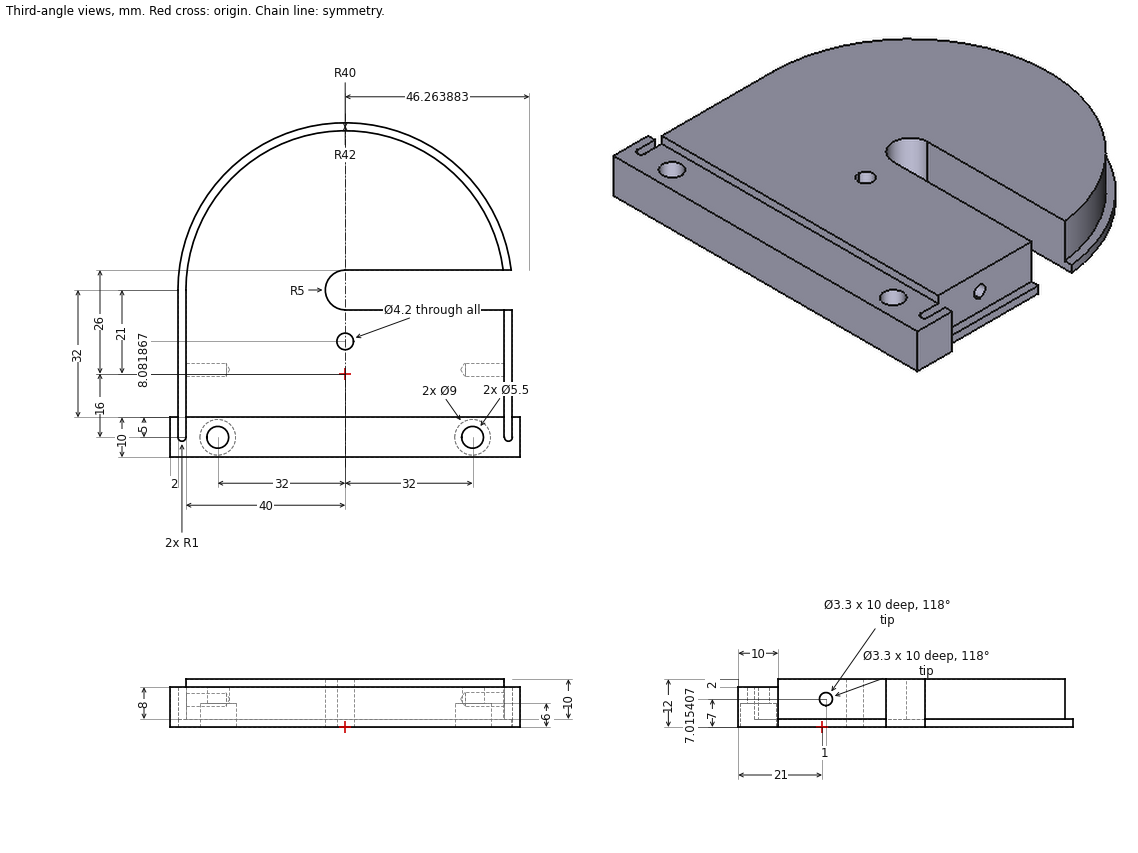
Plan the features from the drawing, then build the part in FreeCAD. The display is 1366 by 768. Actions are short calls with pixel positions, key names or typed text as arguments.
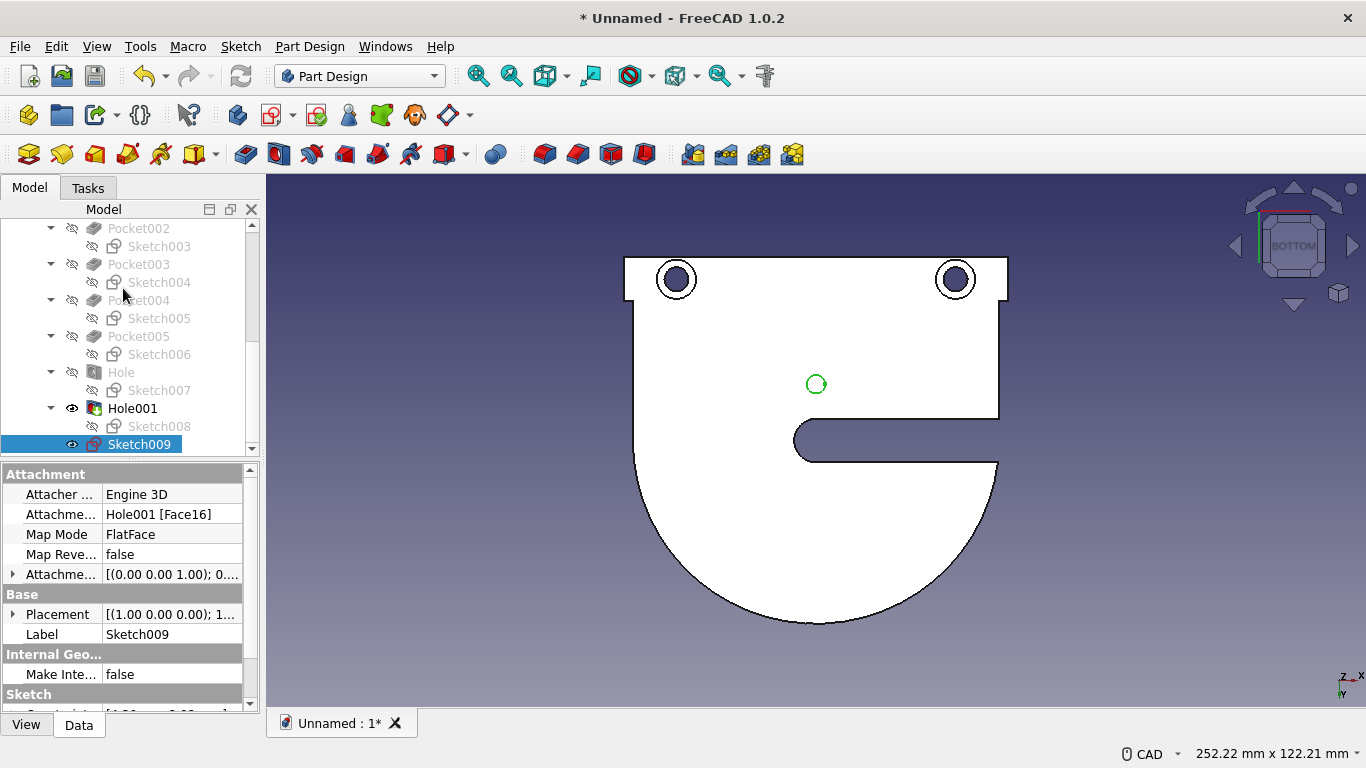
click(279, 154)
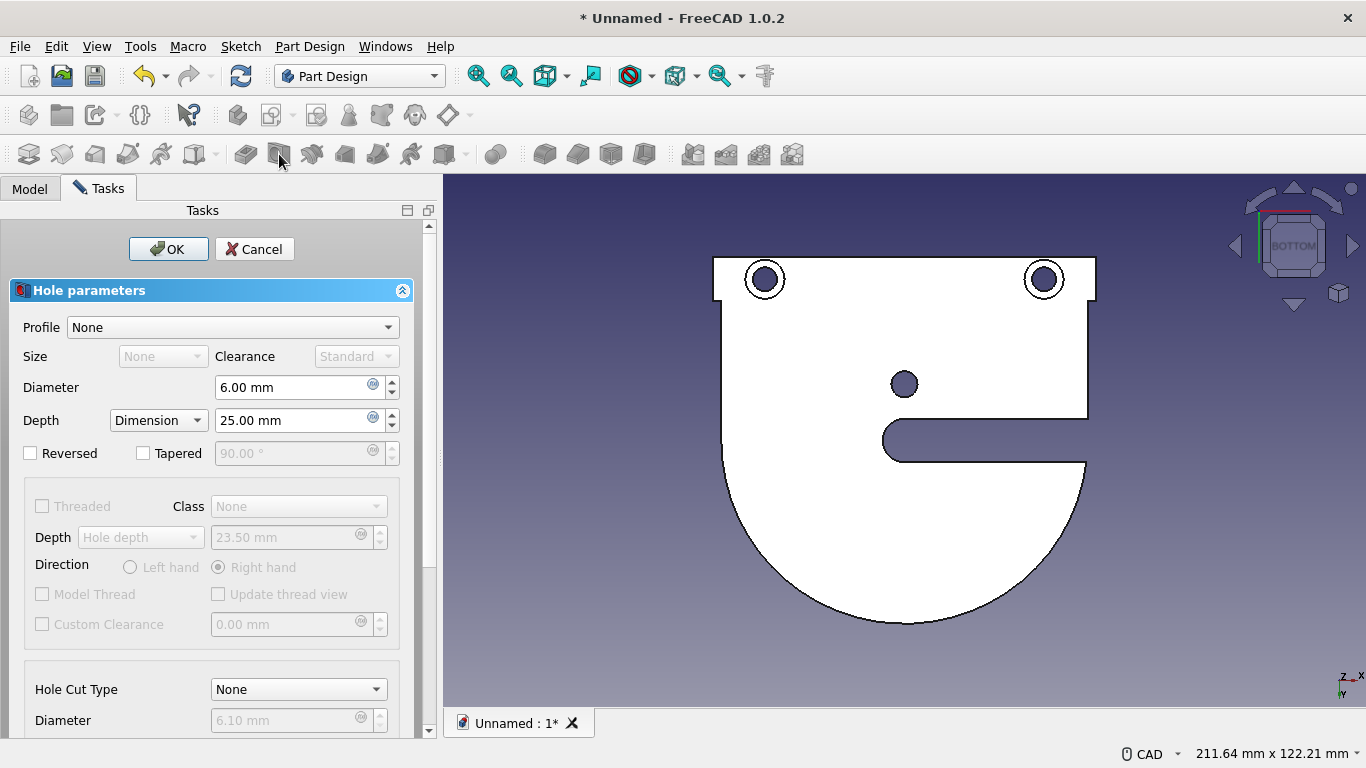
triple_click(300, 388)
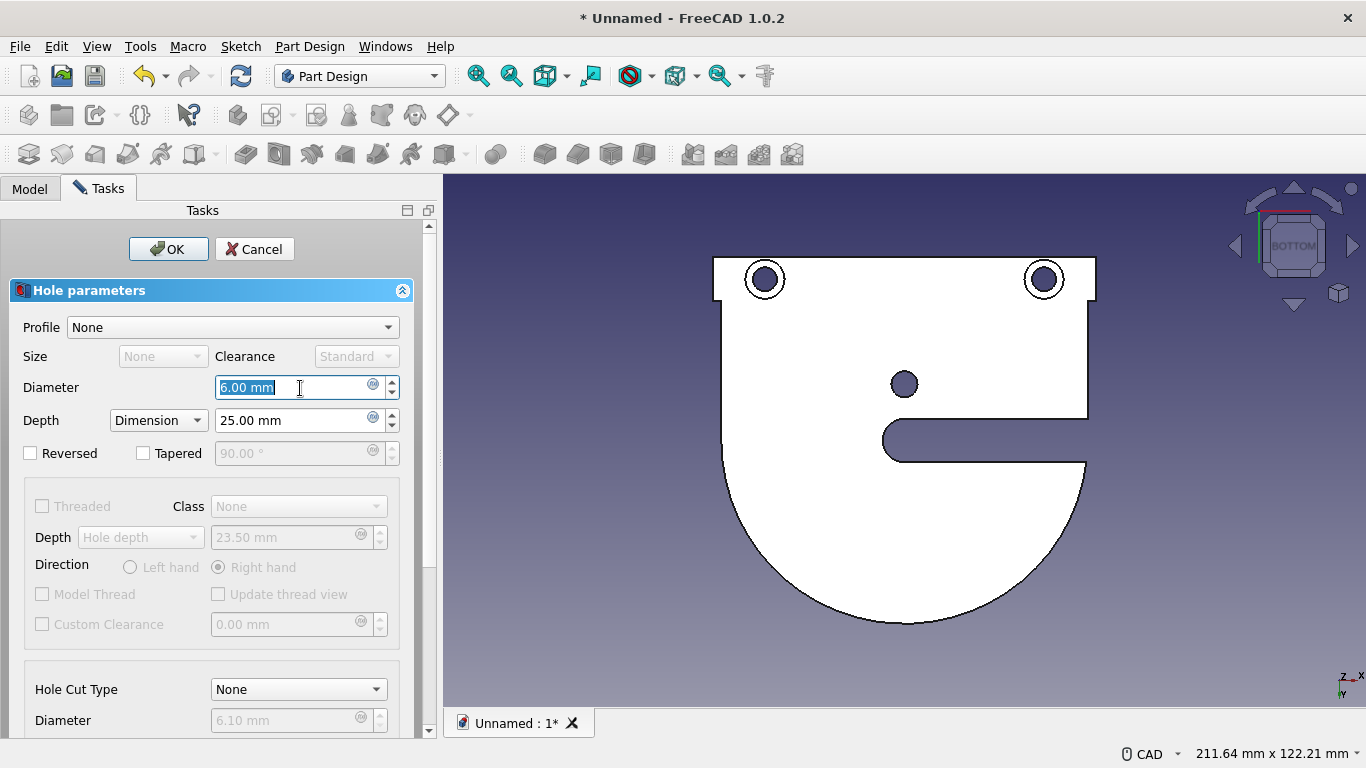
text(4.2)
key(Tab)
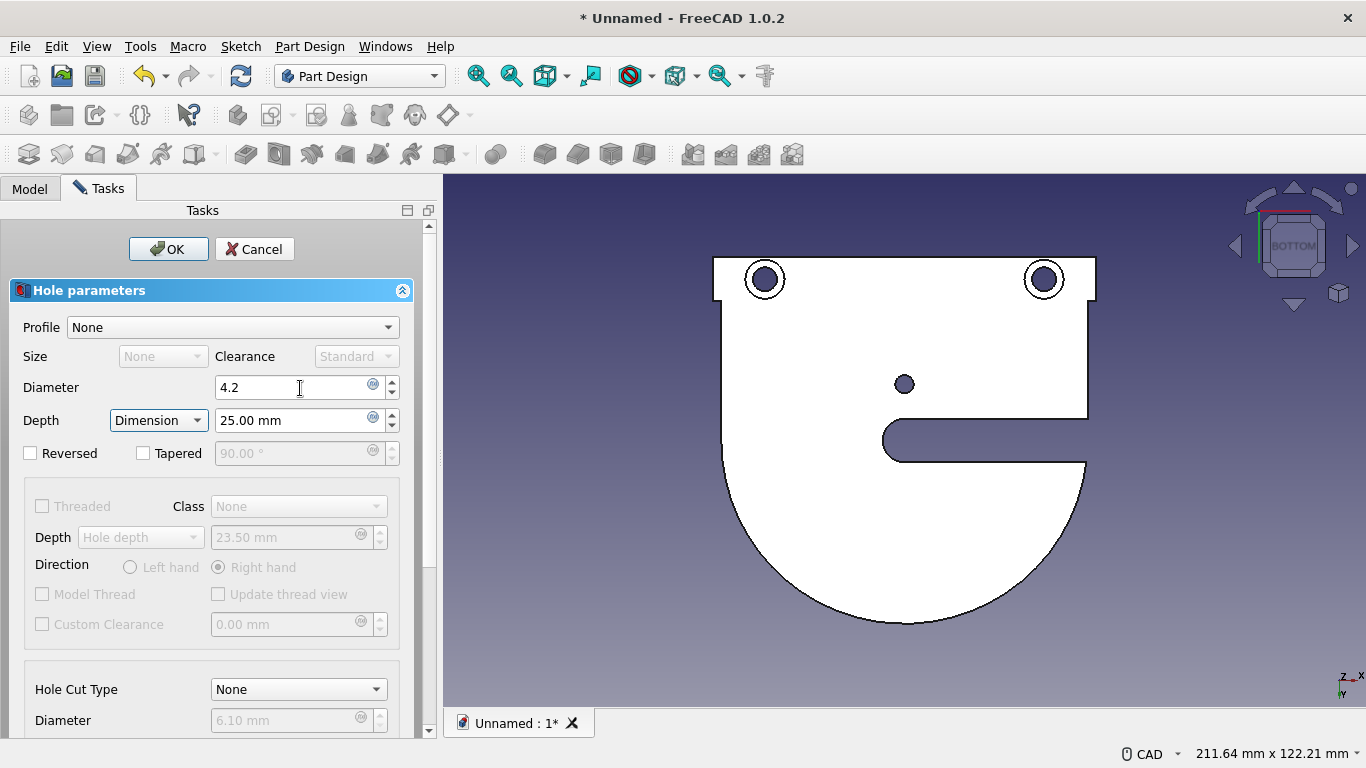
click(160, 420)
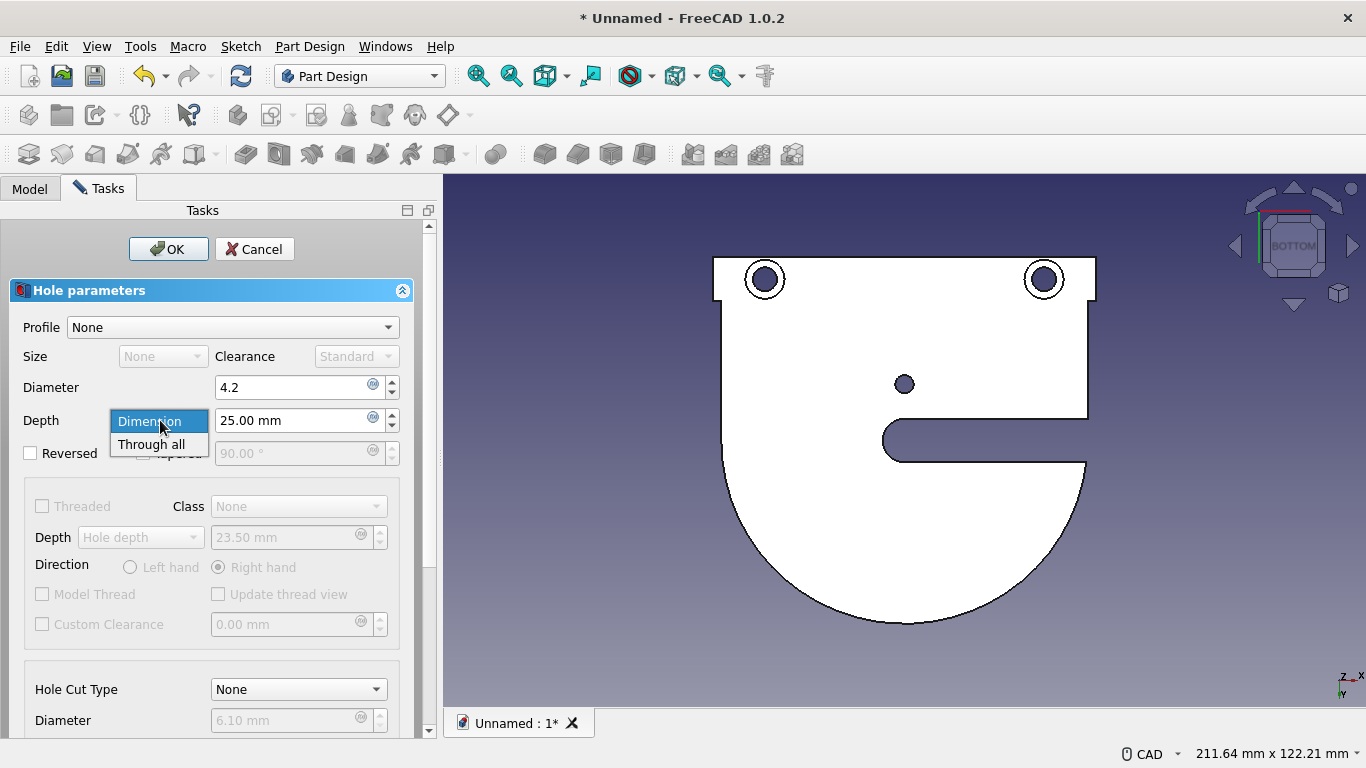
click(158, 444)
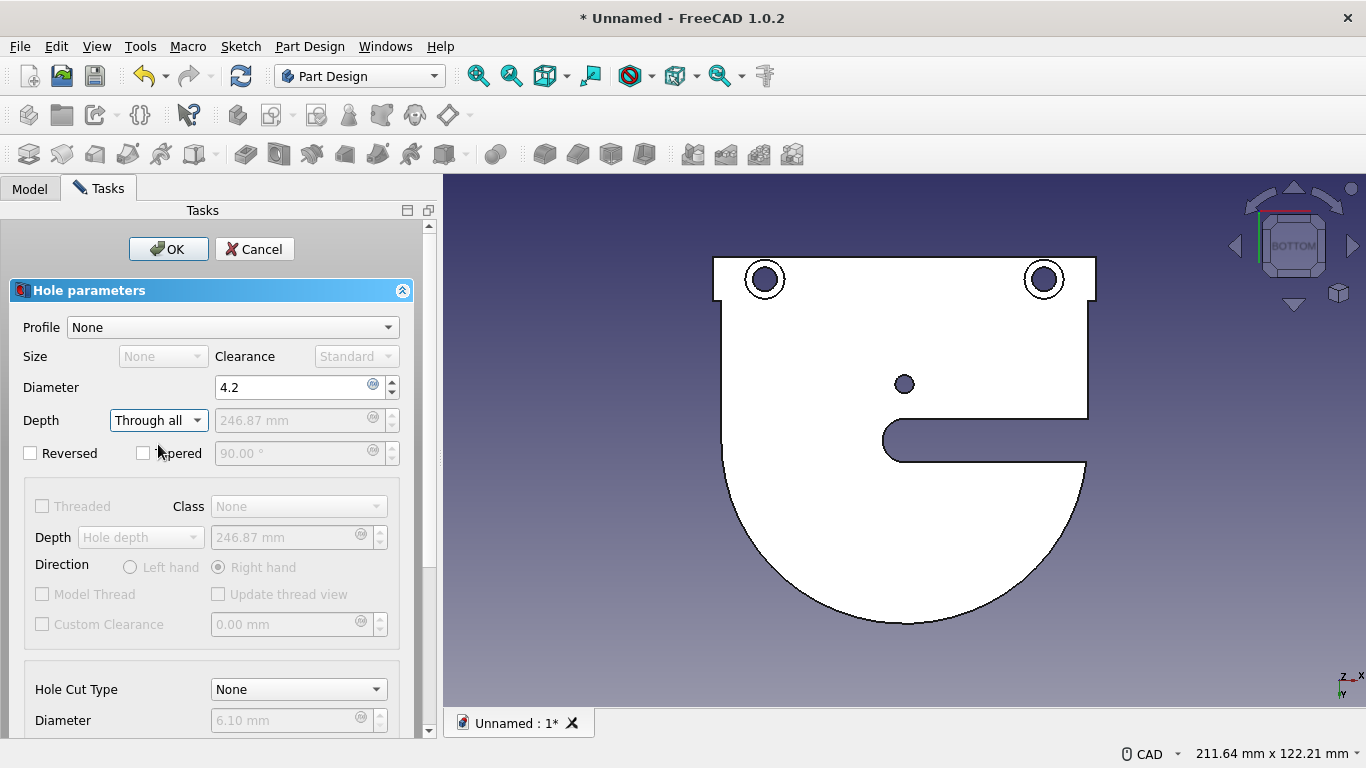
click(169, 249)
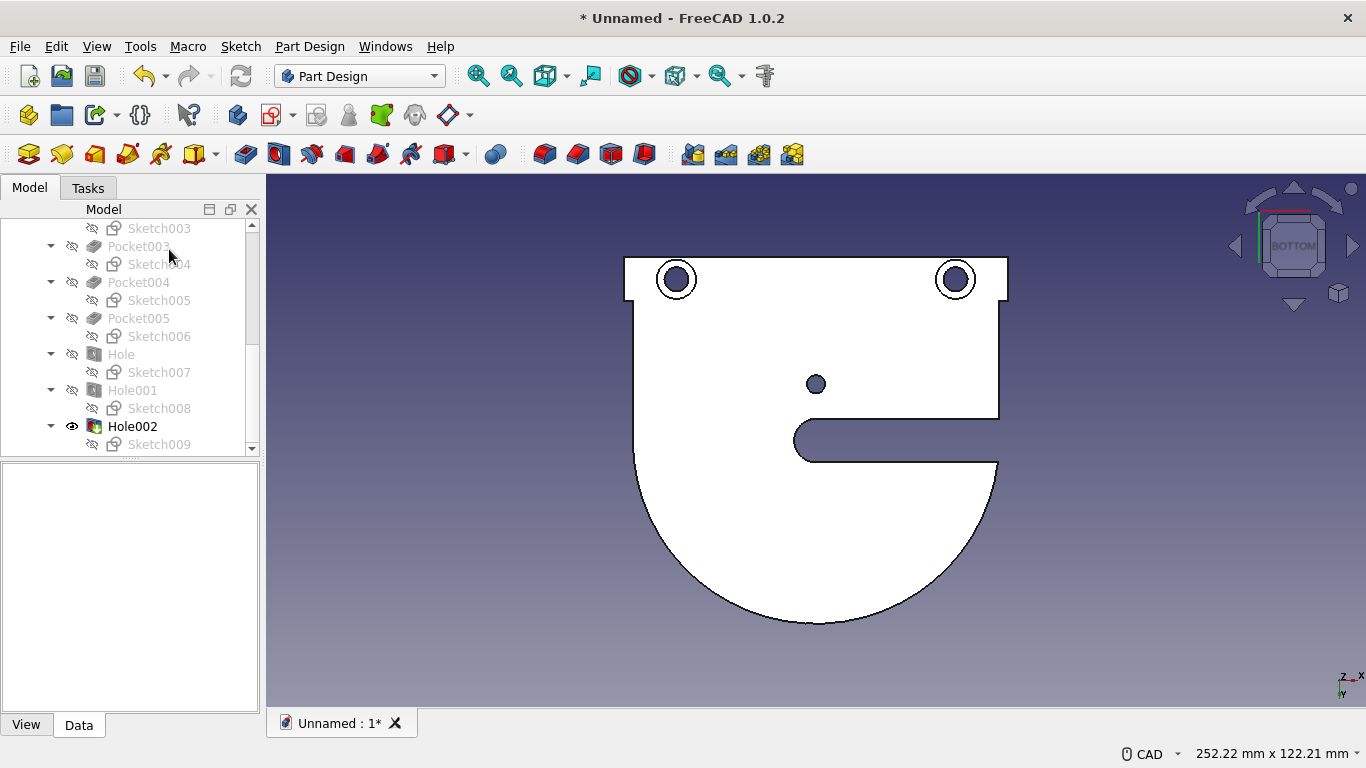
key(0)